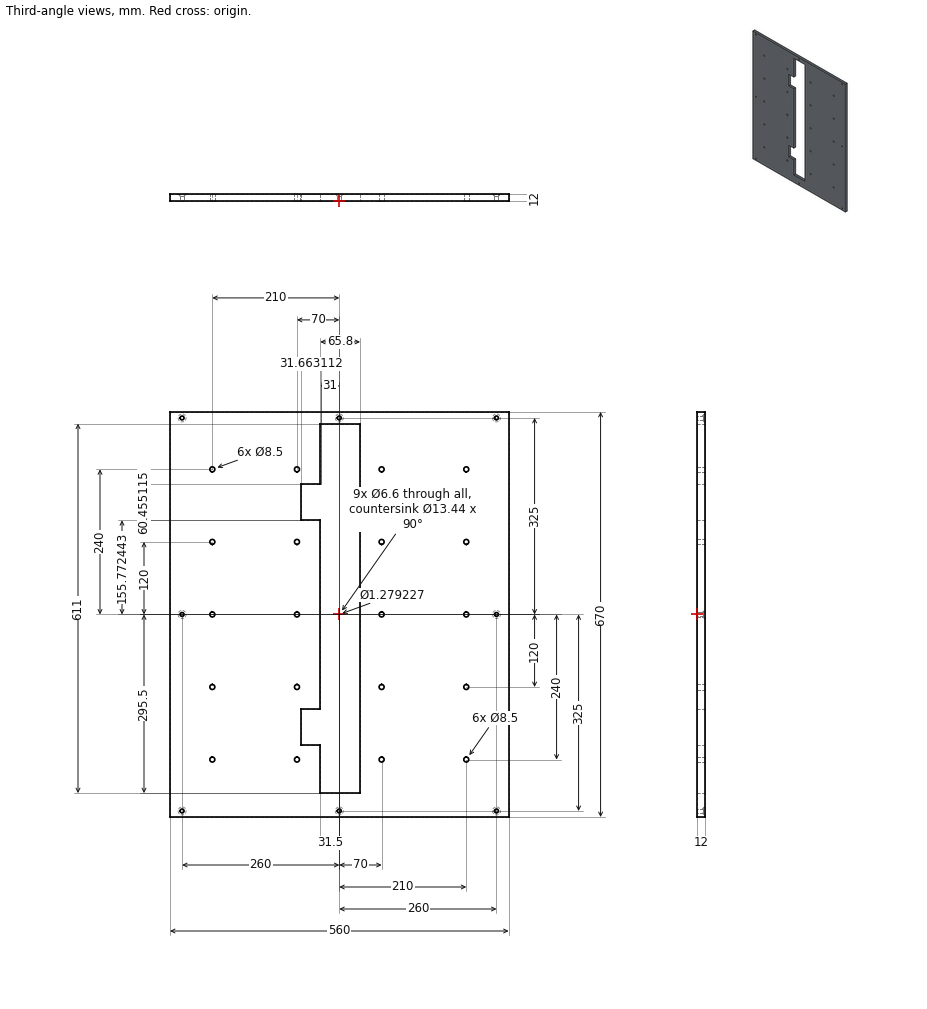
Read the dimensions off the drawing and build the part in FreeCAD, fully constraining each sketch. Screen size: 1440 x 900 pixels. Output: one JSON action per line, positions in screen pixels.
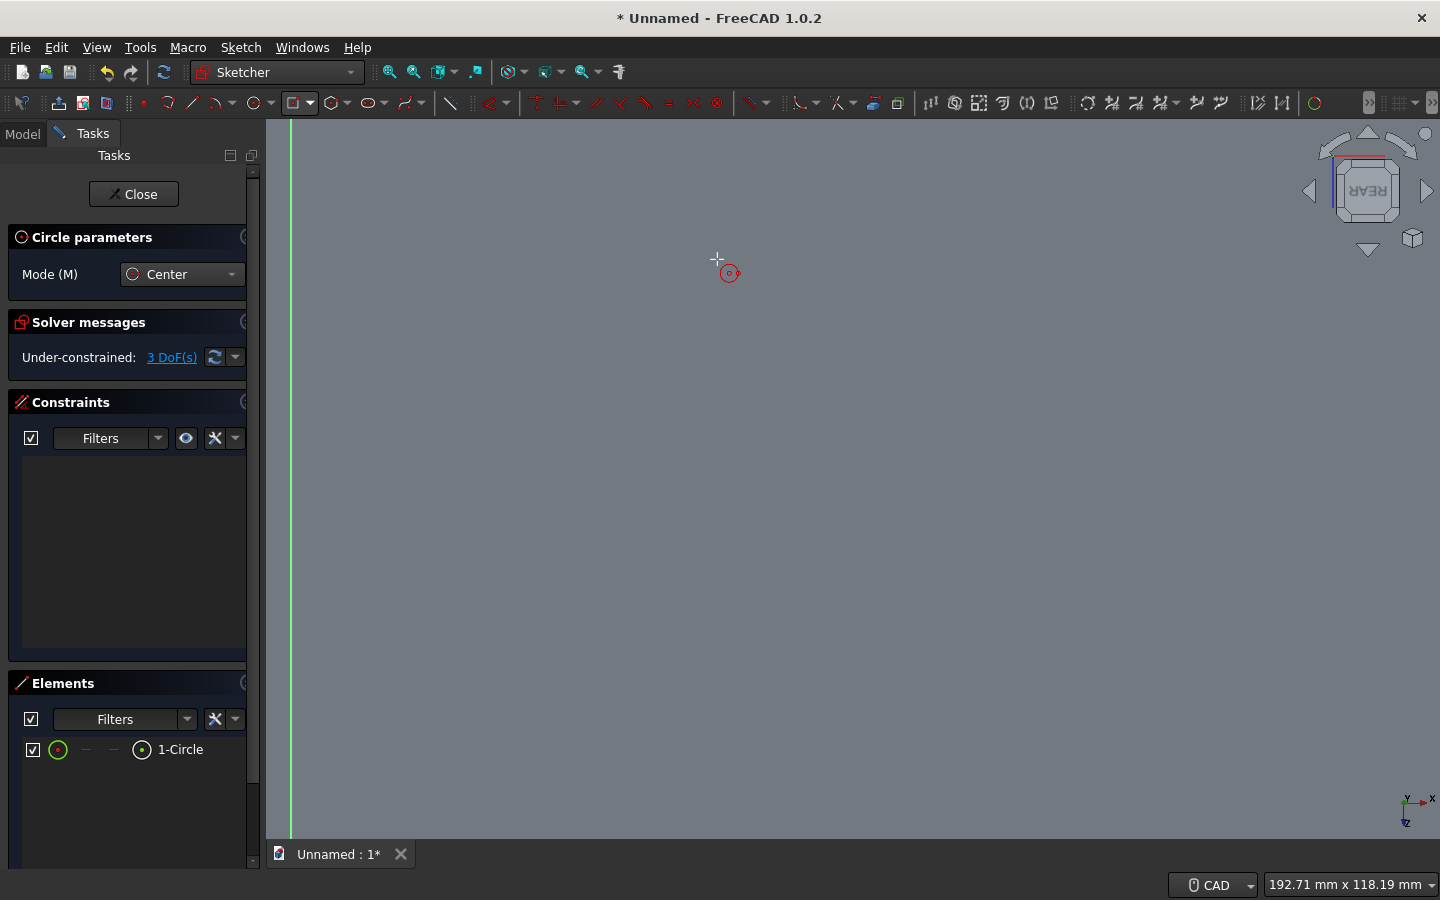
{"action": "left_click", "coordinate": [717, 258]}
{"action": "left_click", "coordinate": [735, 240]}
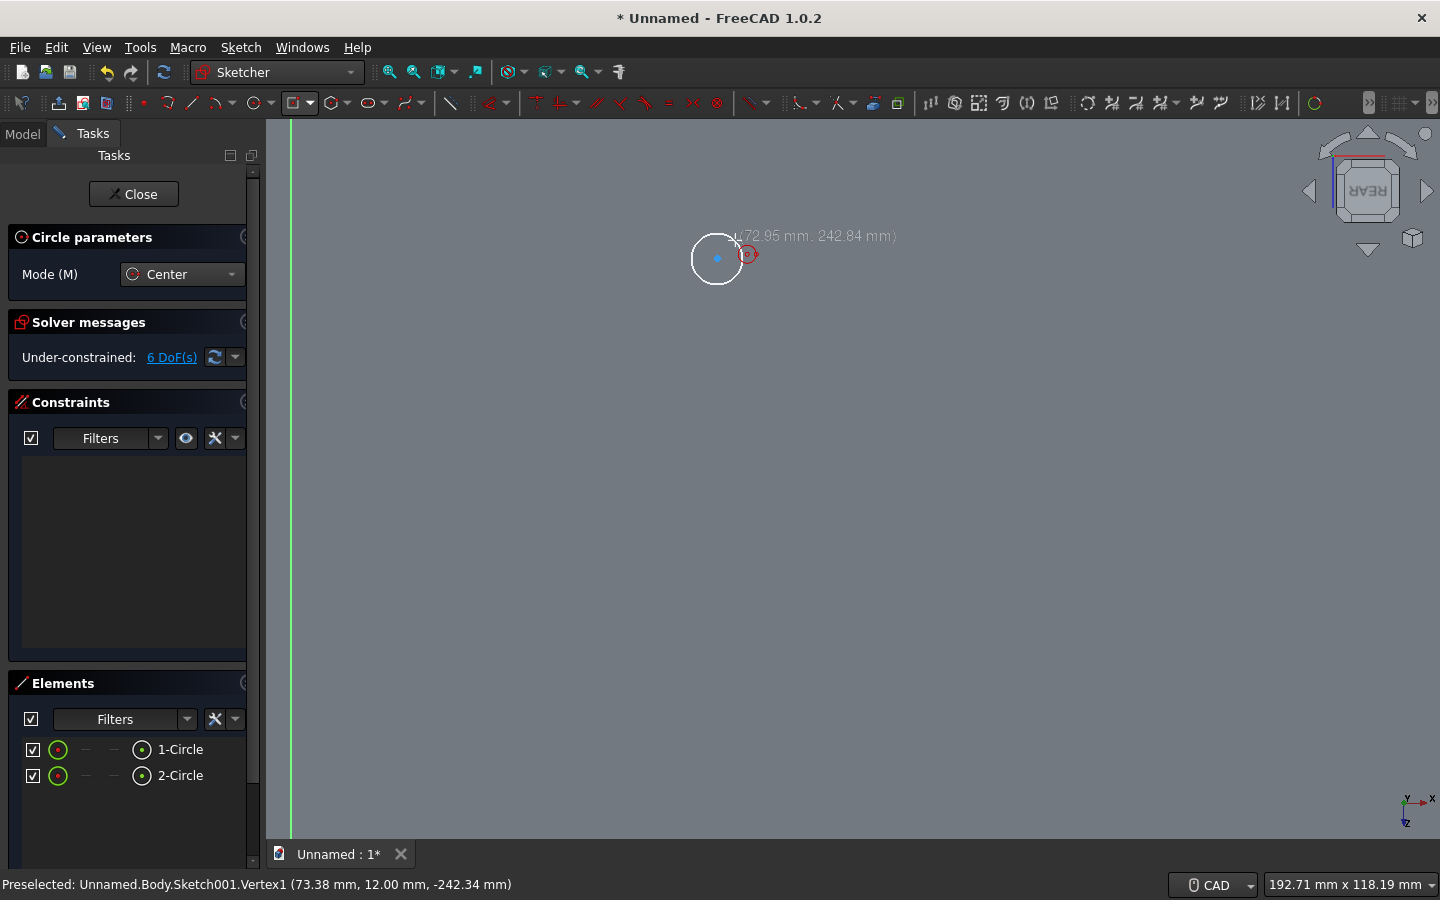
{"action": "scroll", "coordinate": [717, 259], "scroll_direction": "down", "scroll_amount": 6}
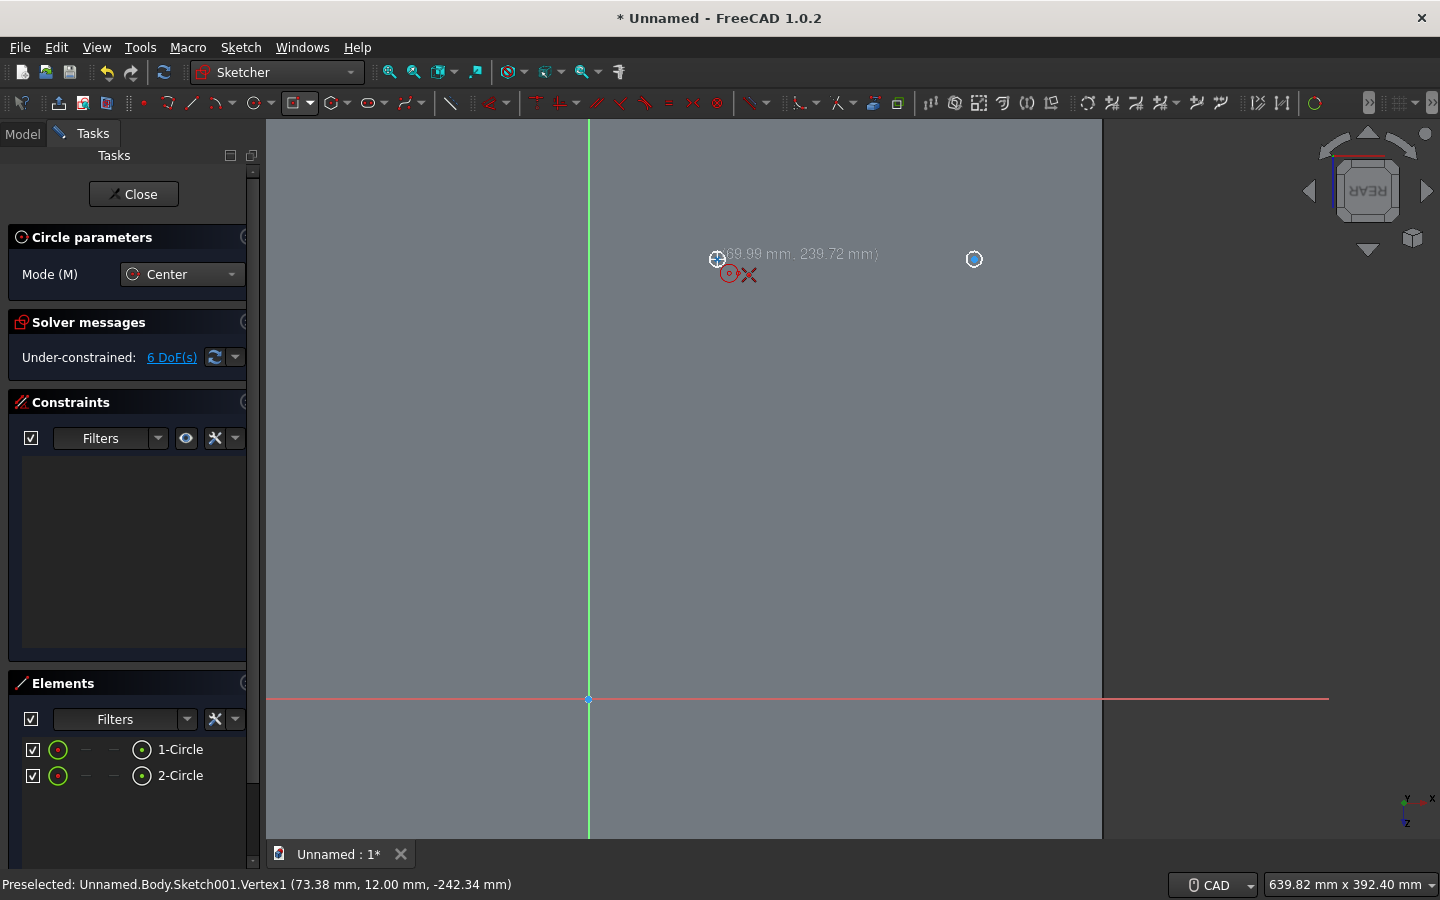
{"action": "scroll", "coordinate": [974, 479], "scroll_direction": "up", "scroll_amount": 6}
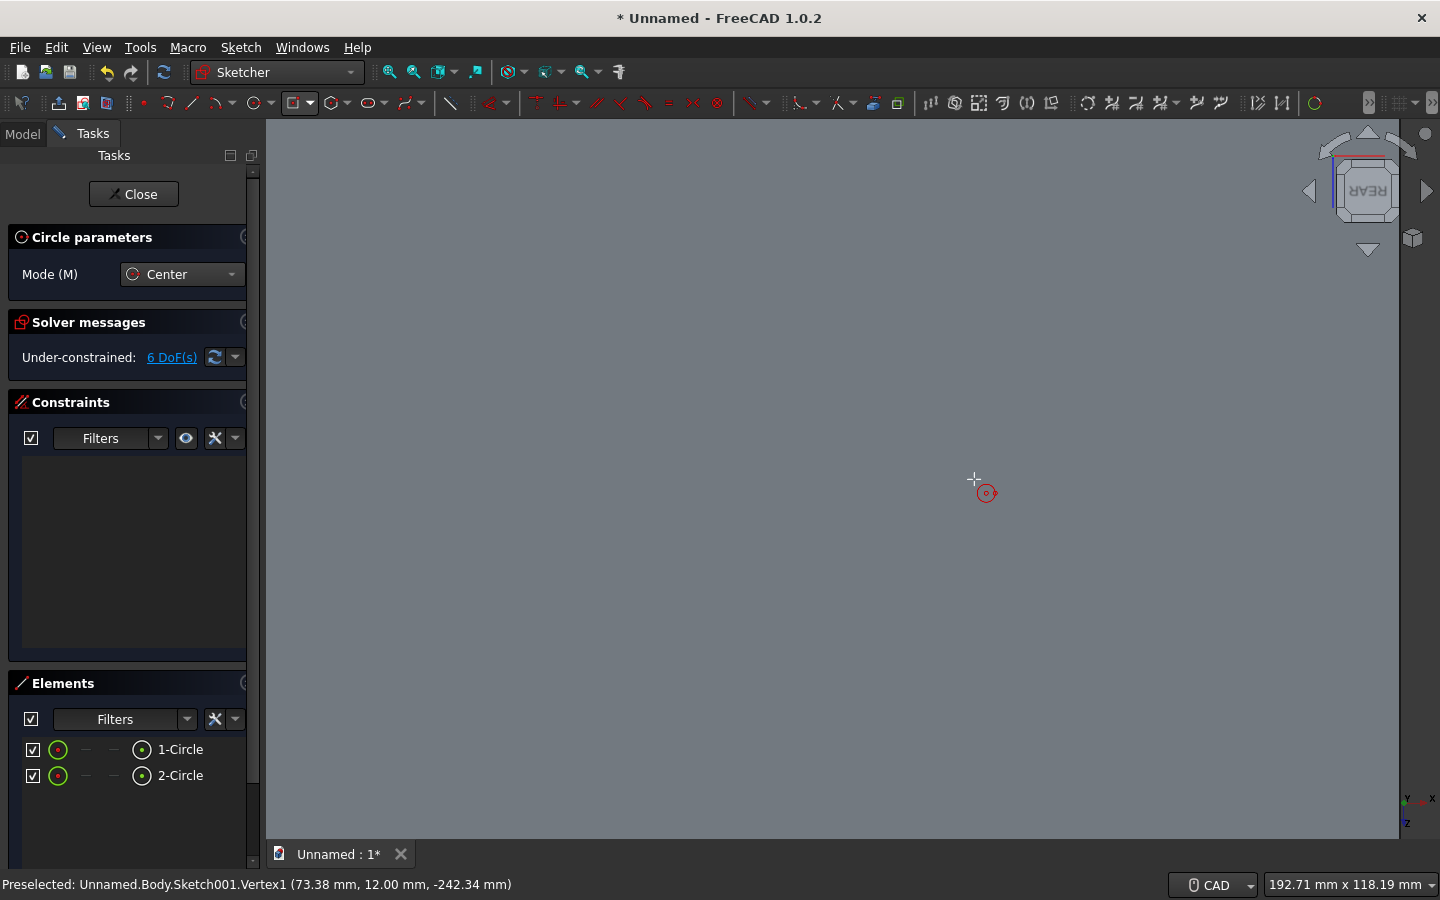
{"action": "left_click", "coordinate": [973, 478]}
{"action": "left_click", "coordinate": [991, 460]}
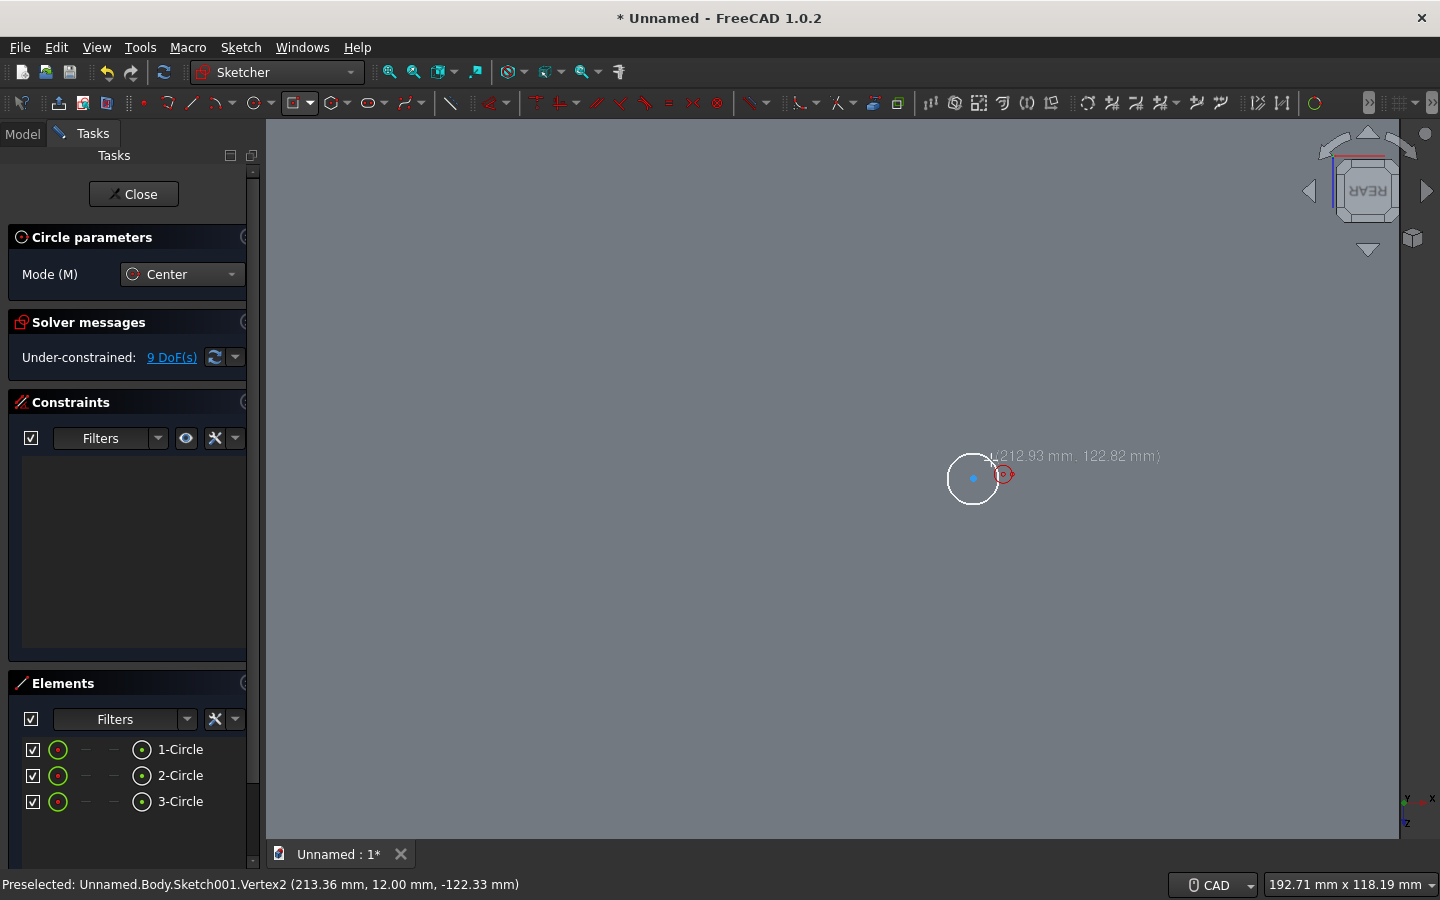
{"action": "scroll", "coordinate": [974, 479], "scroll_direction": "down", "scroll_amount": 6}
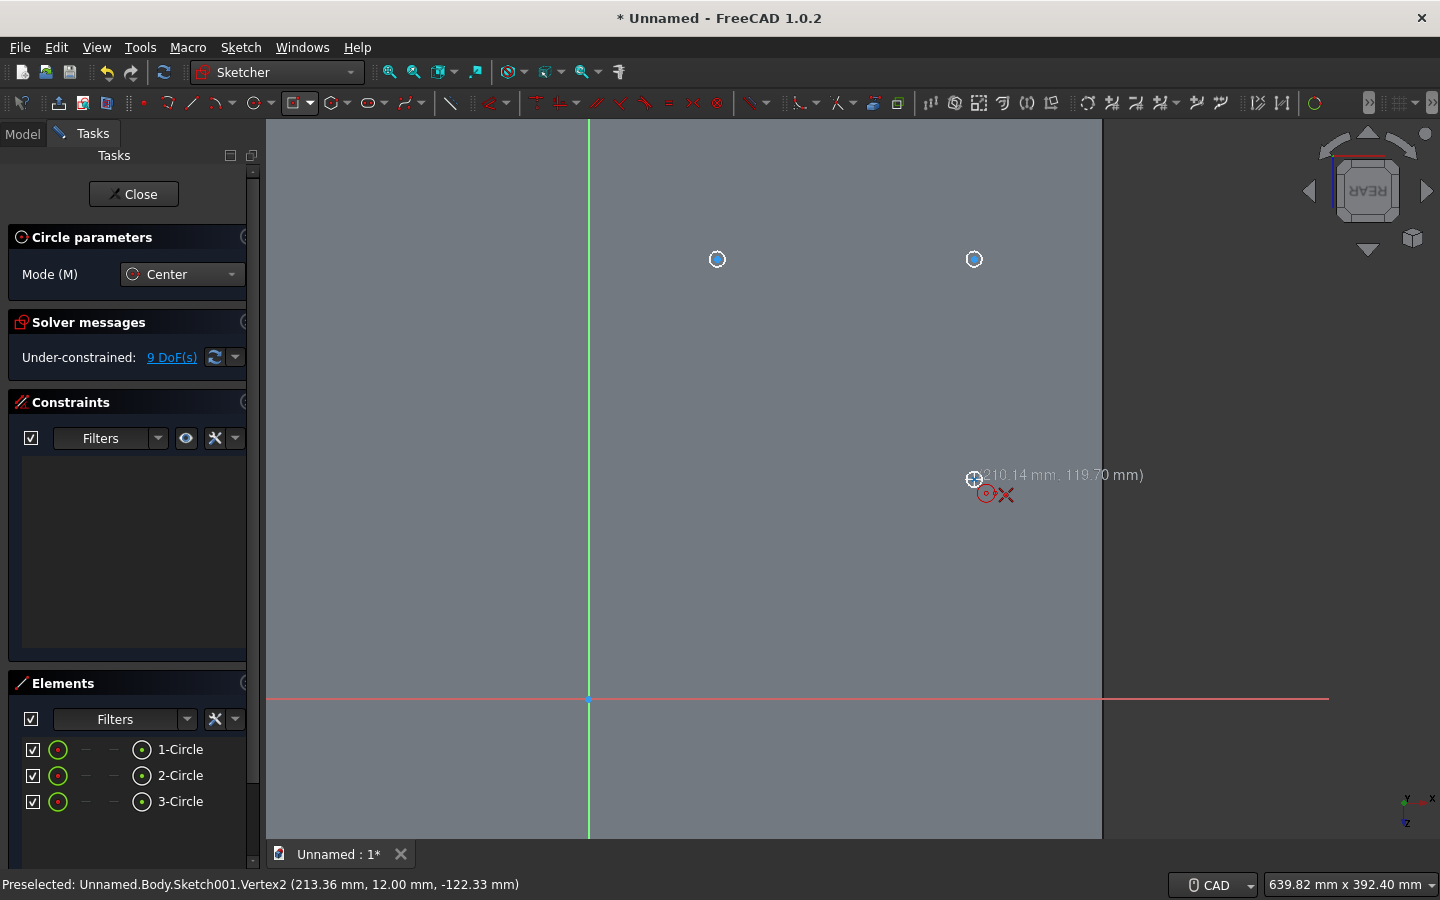
{"action": "scroll", "coordinate": [717, 479], "scroll_direction": "up", "scroll_amount": 6}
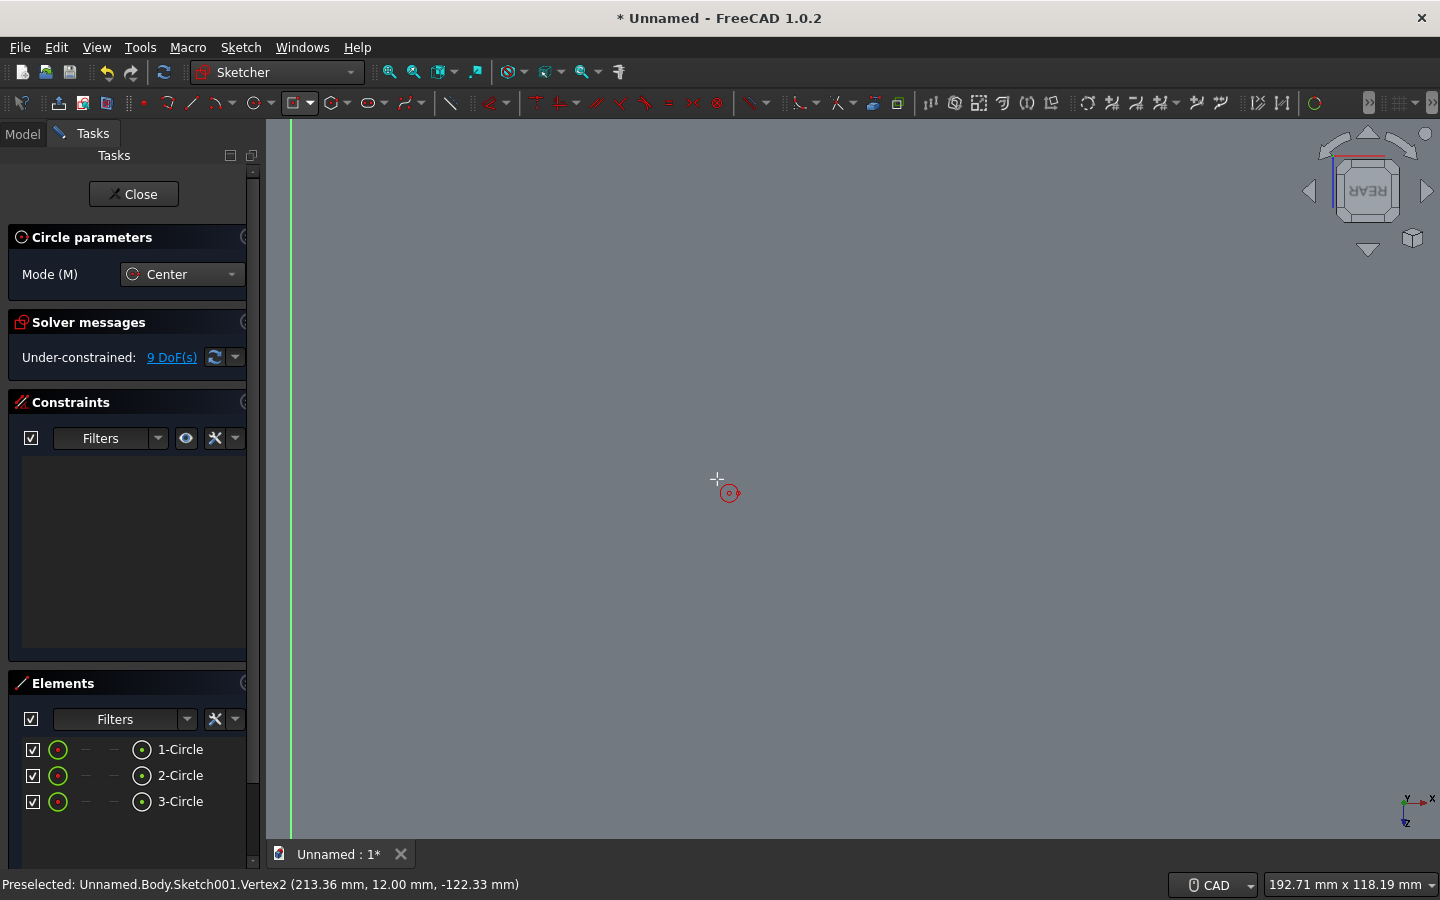
{"action": "left_click", "coordinate": [717, 478]}
{"action": "left_click", "coordinate": [735, 460]}